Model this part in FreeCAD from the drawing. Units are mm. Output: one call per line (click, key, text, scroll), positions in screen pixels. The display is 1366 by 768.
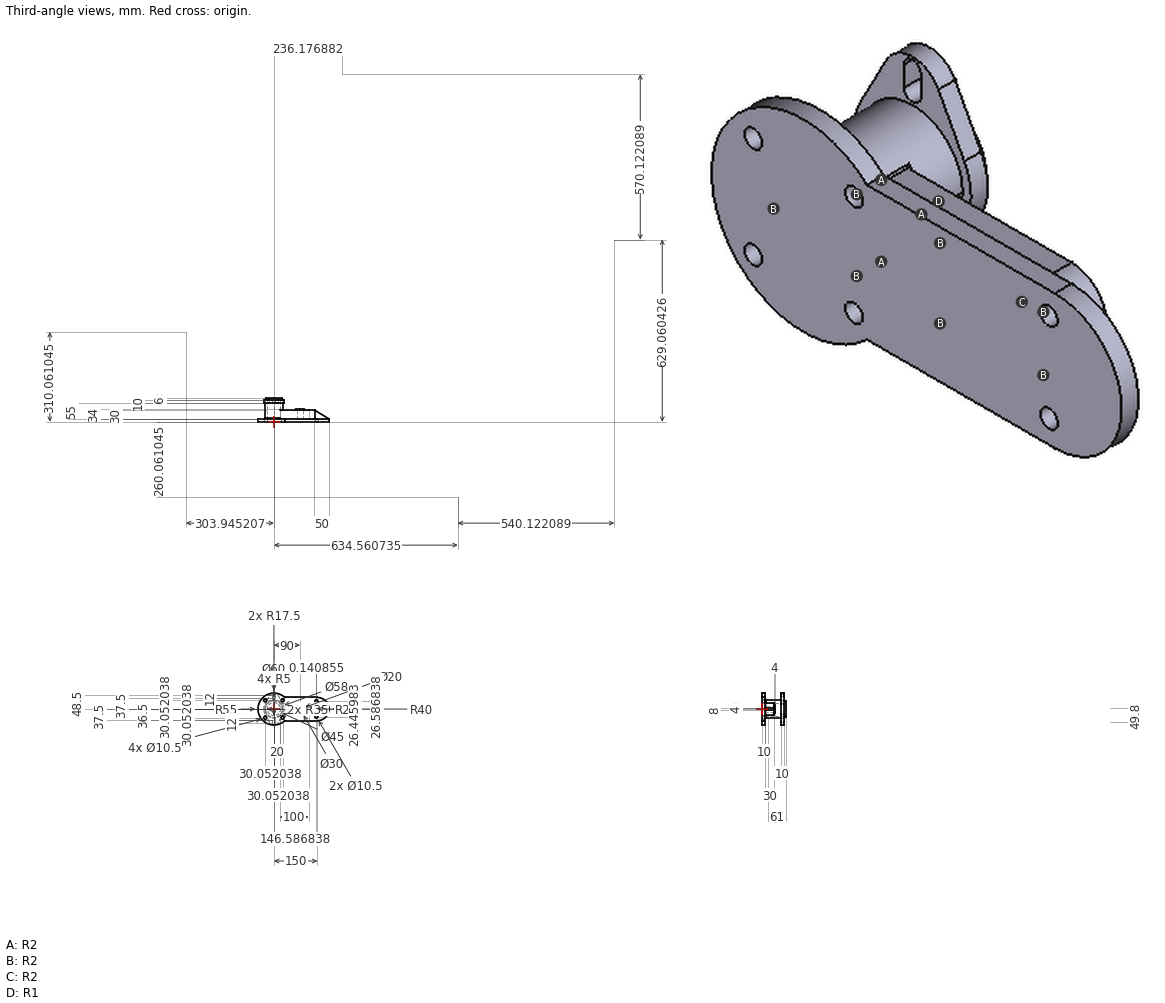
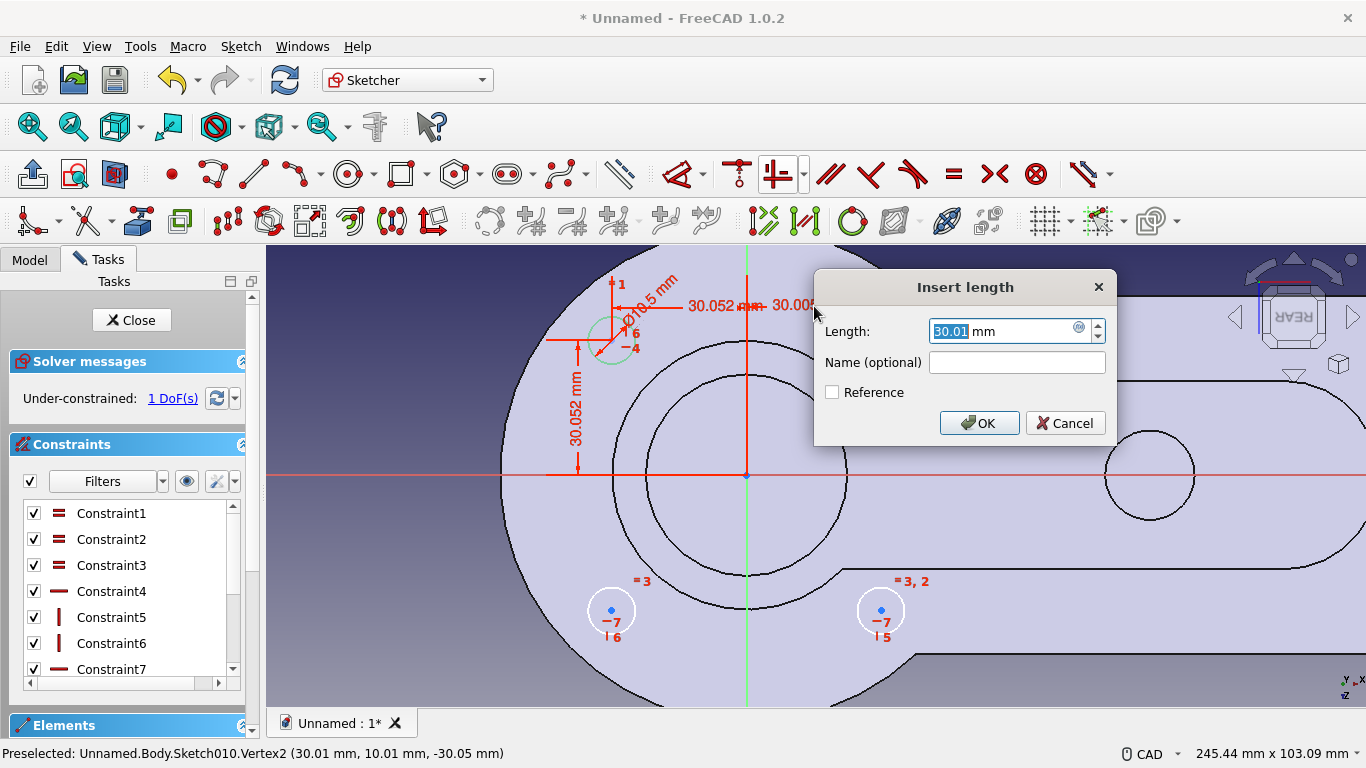
text(30.052038)
key(Return)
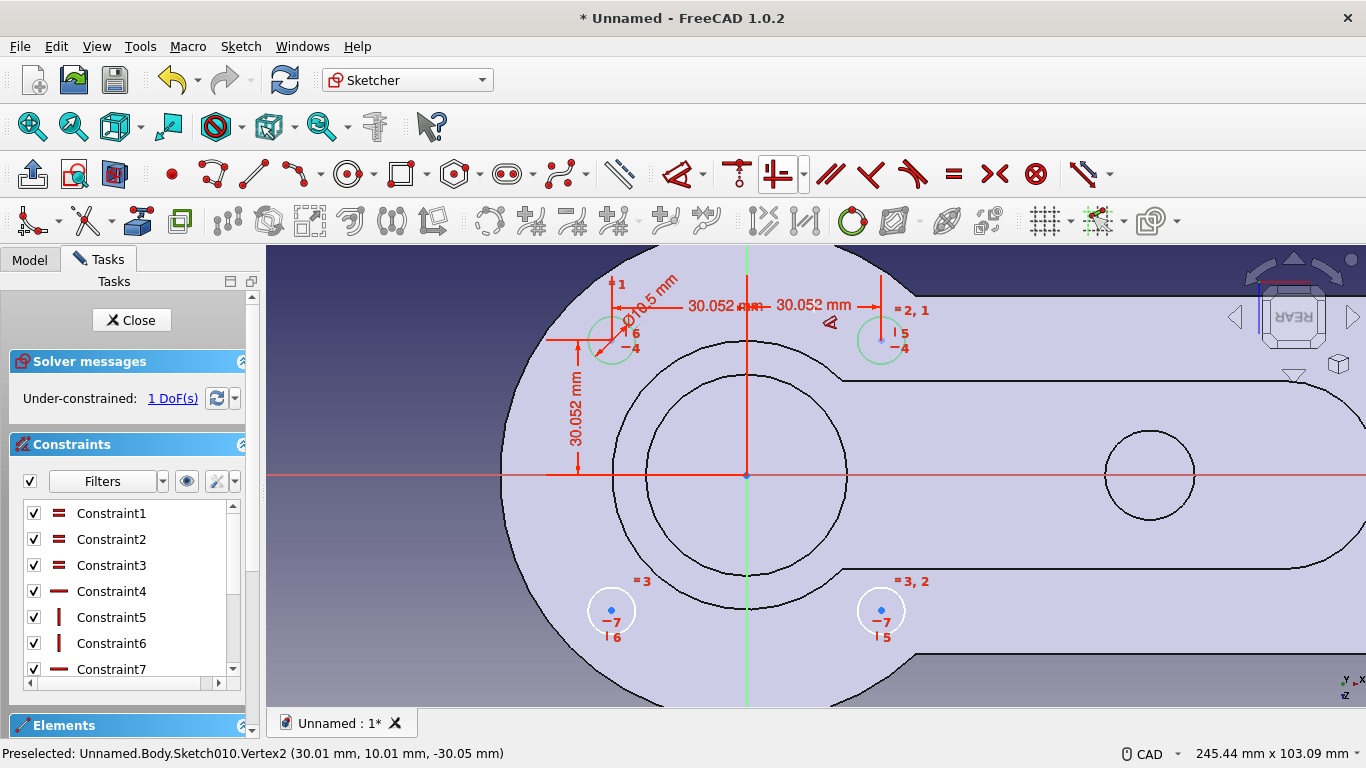
click(881, 611)
click(915, 543)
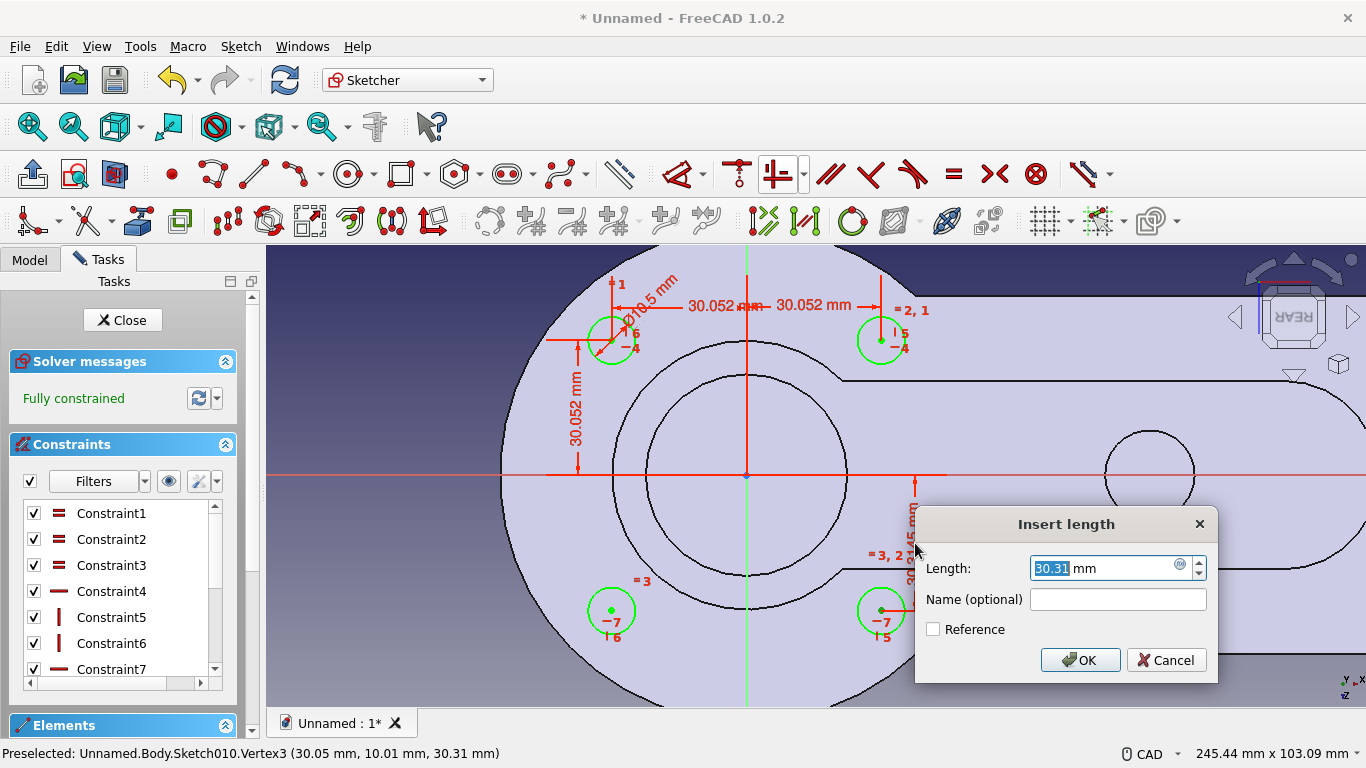
text(30.052038)
key(Return)
key(Escape)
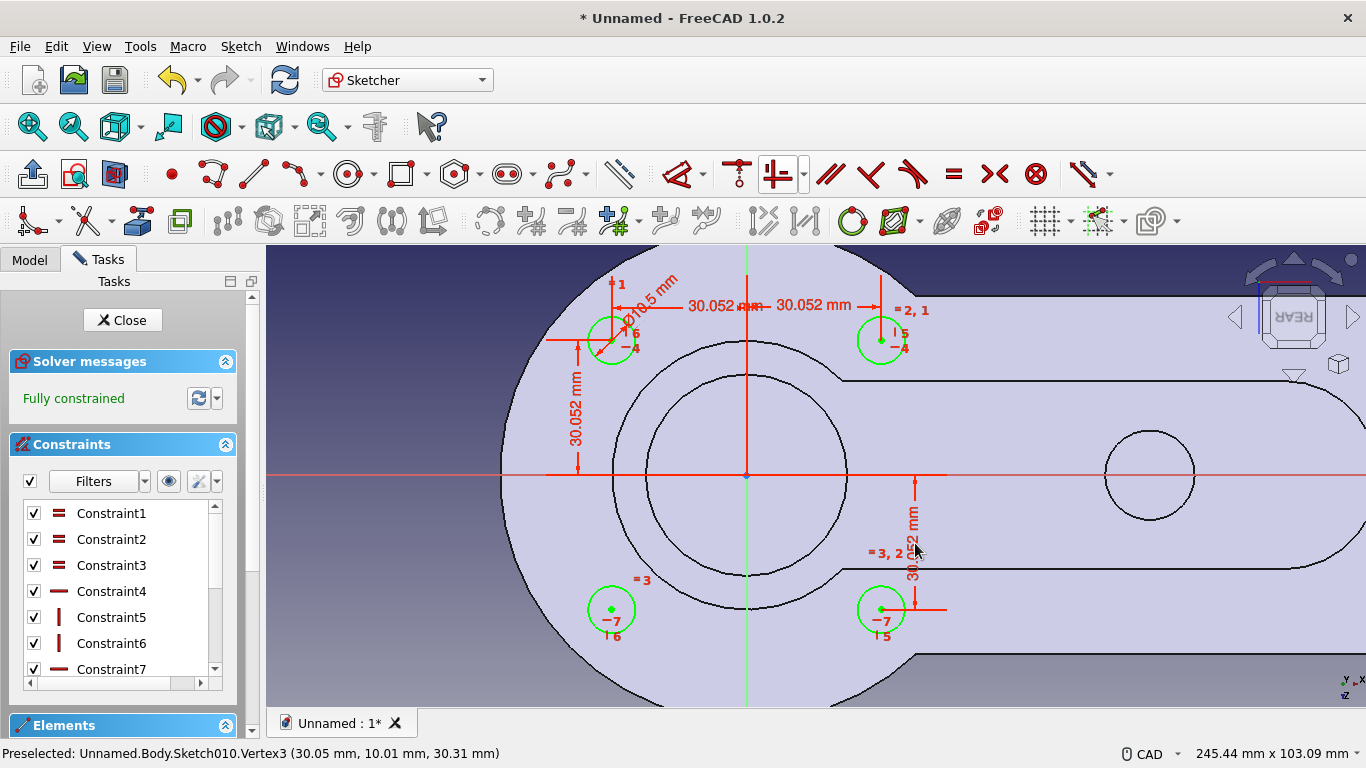
click(123, 320)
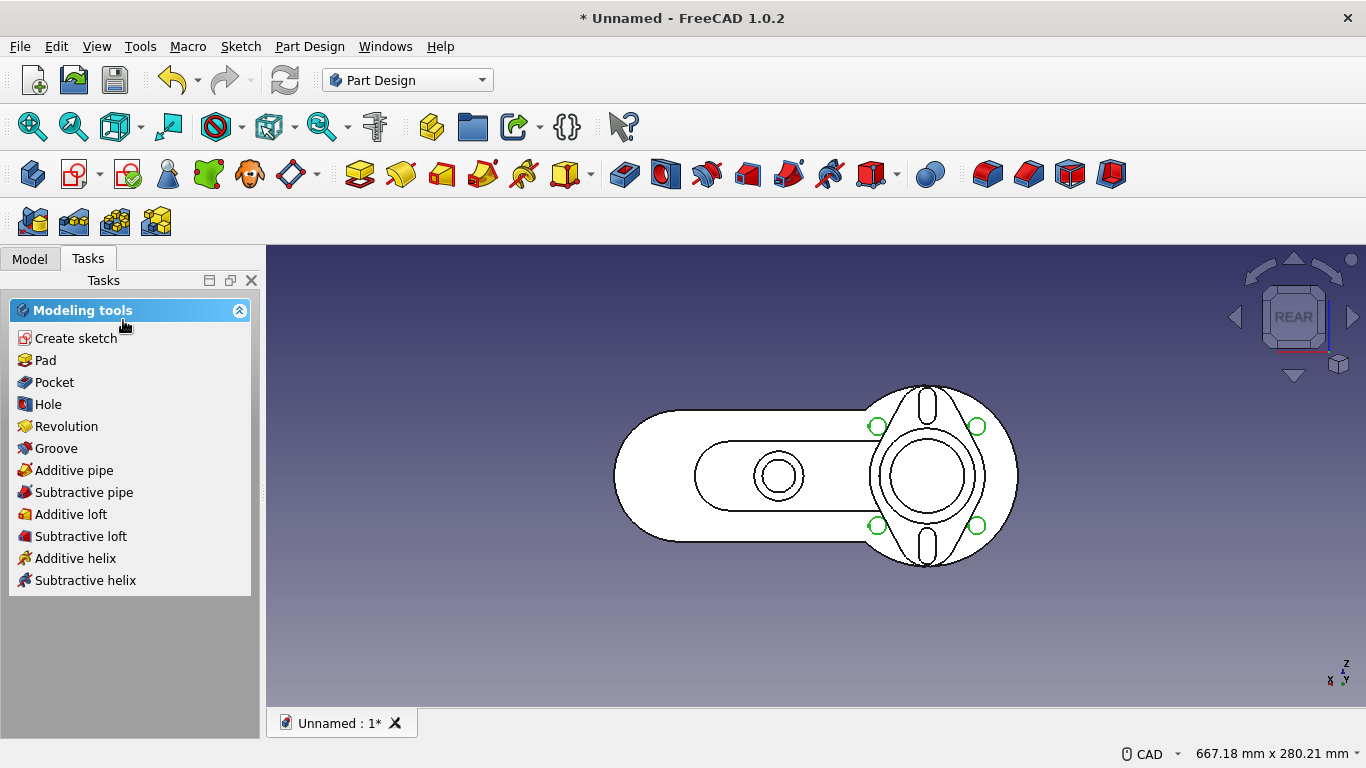
click(625, 174)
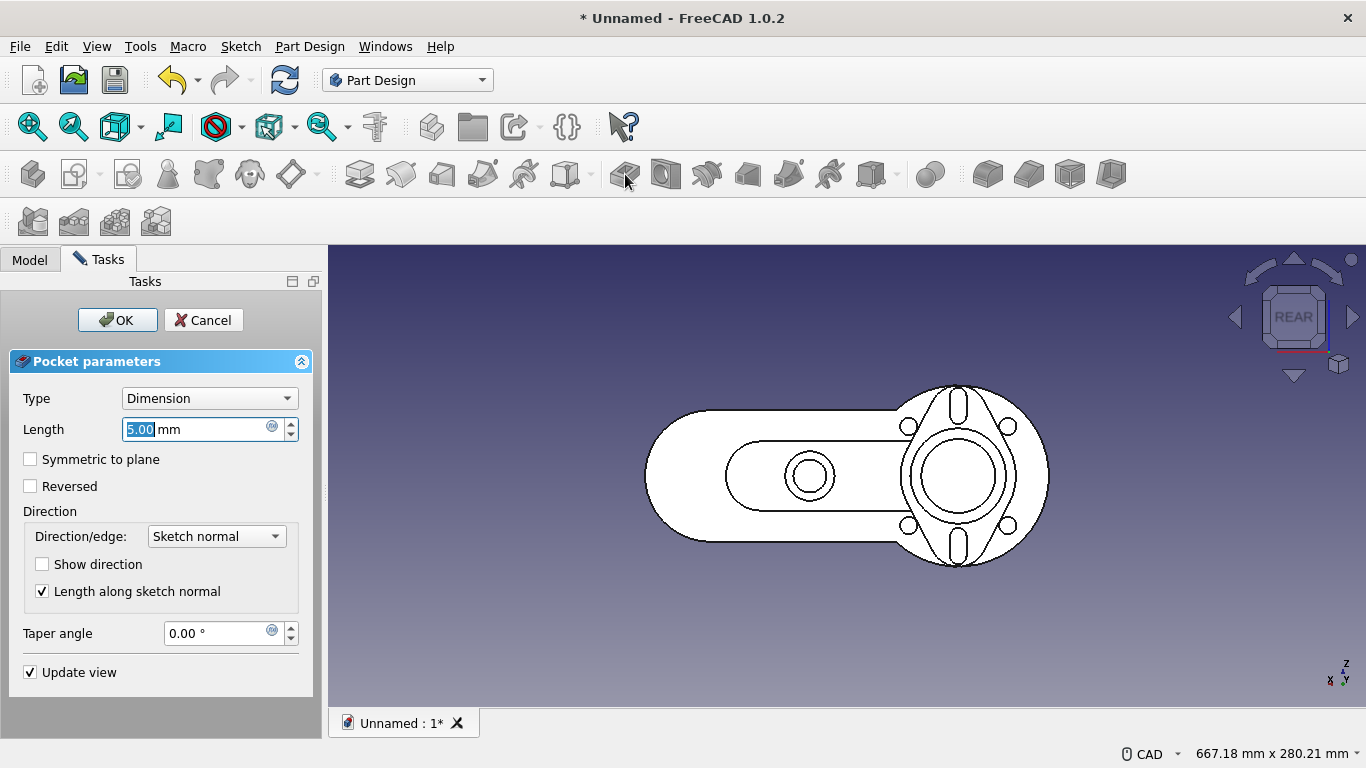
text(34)
key(Tab)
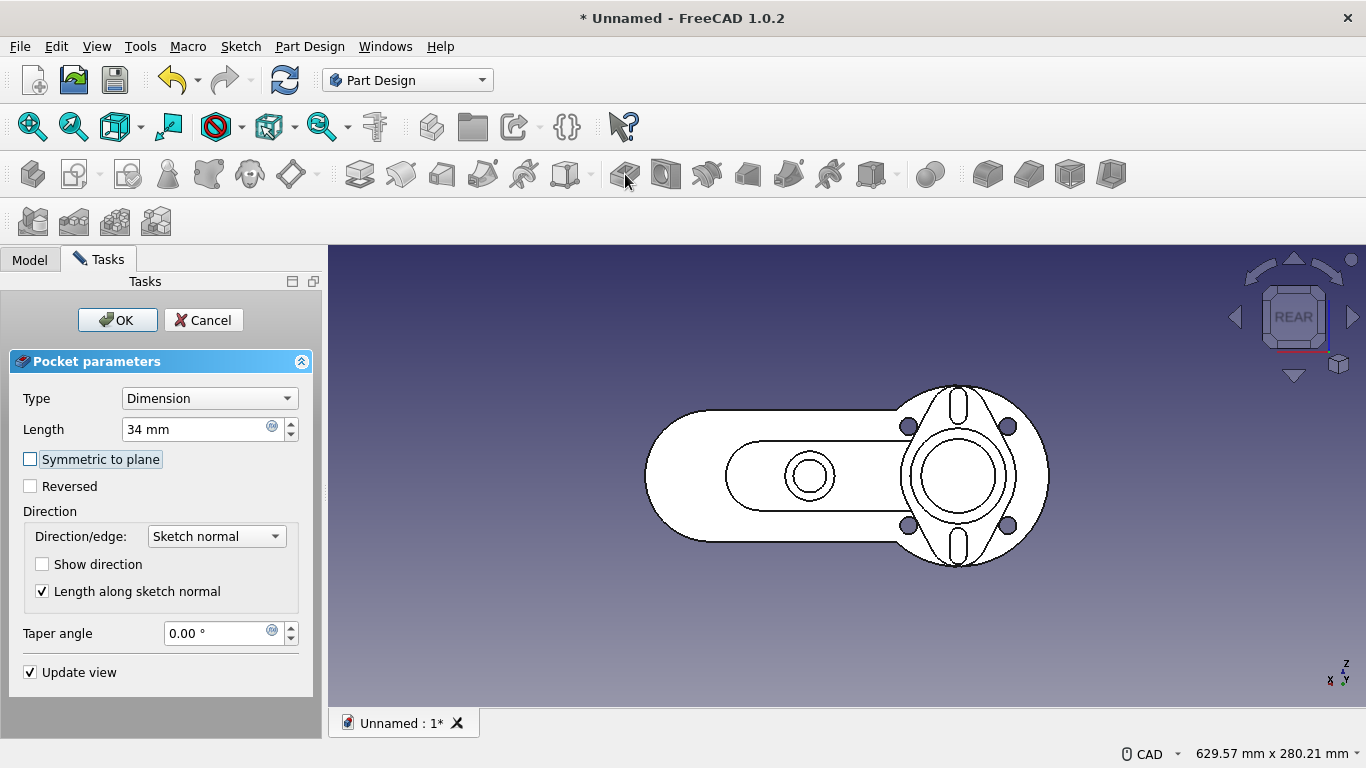
click(118, 320)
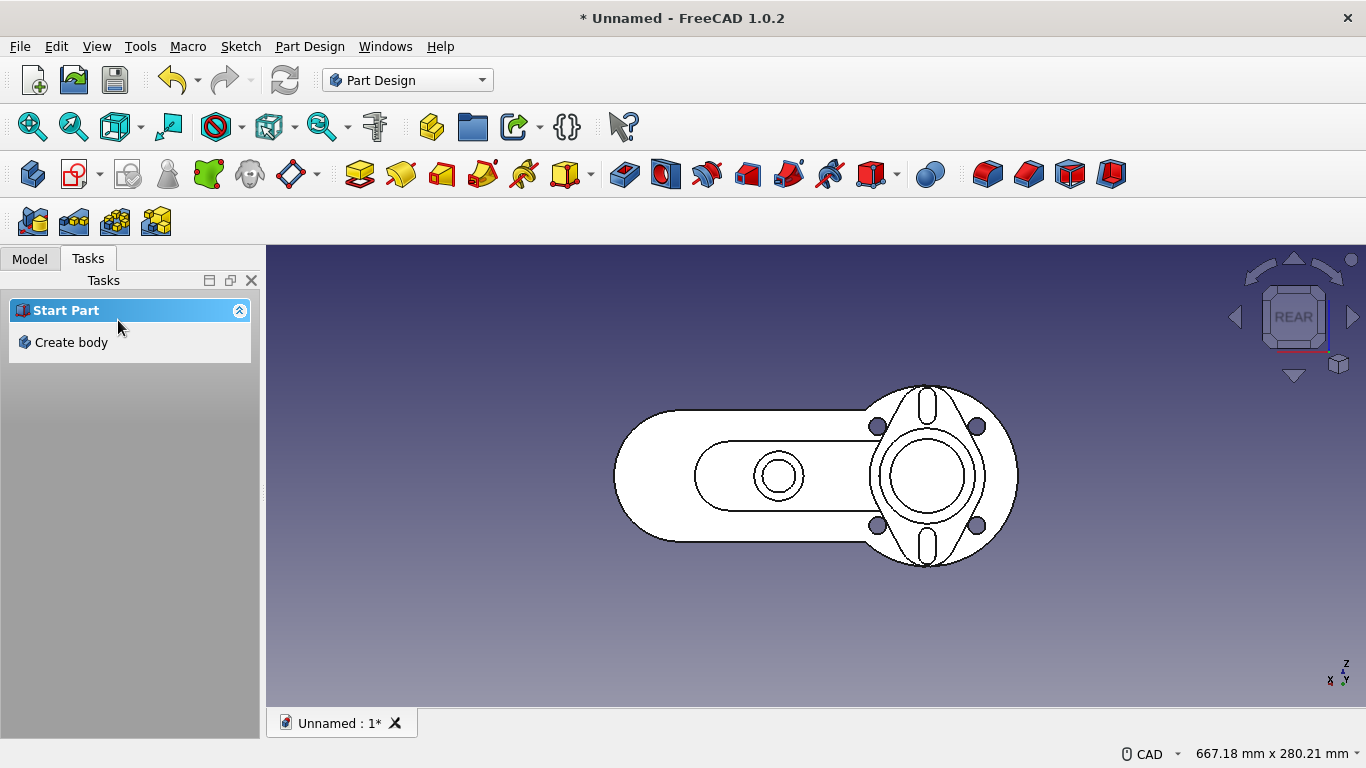
key(v)
key(f)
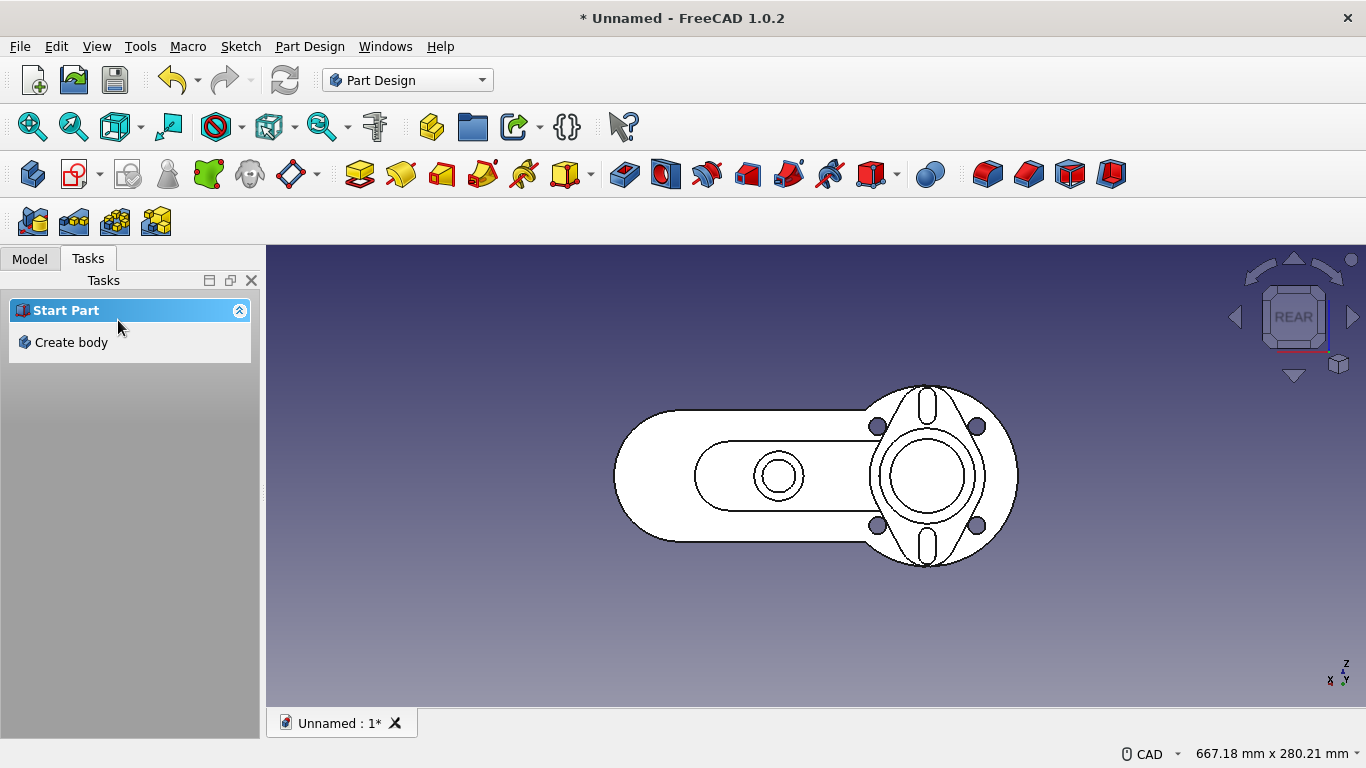
click(643, 475)